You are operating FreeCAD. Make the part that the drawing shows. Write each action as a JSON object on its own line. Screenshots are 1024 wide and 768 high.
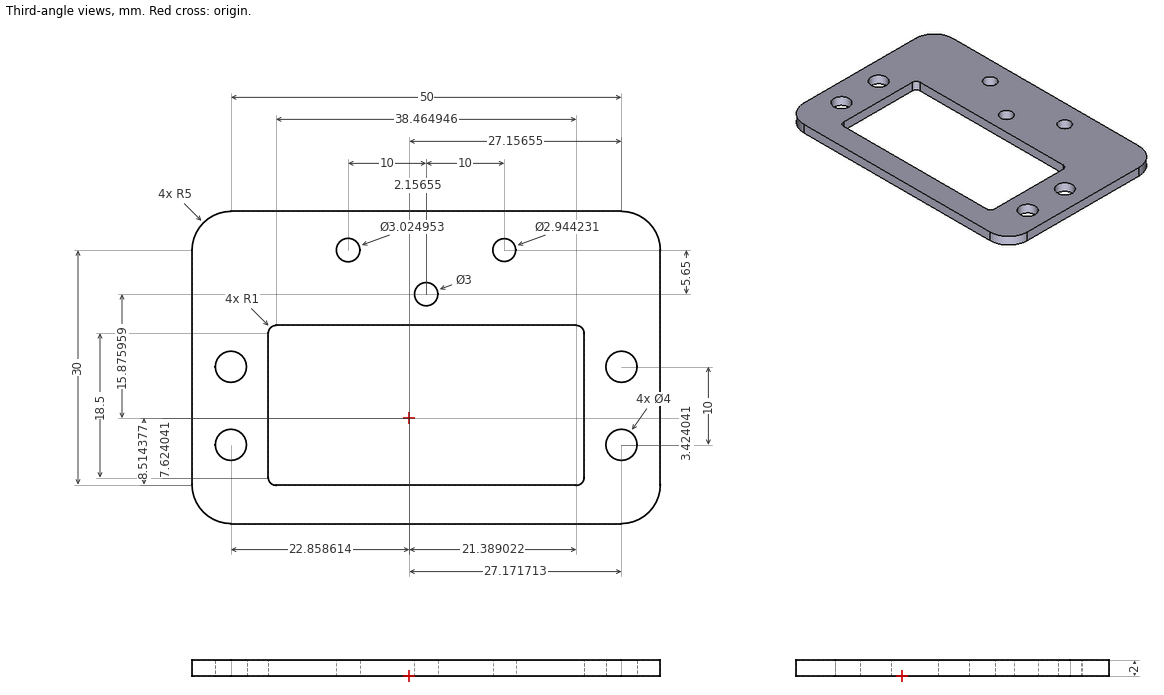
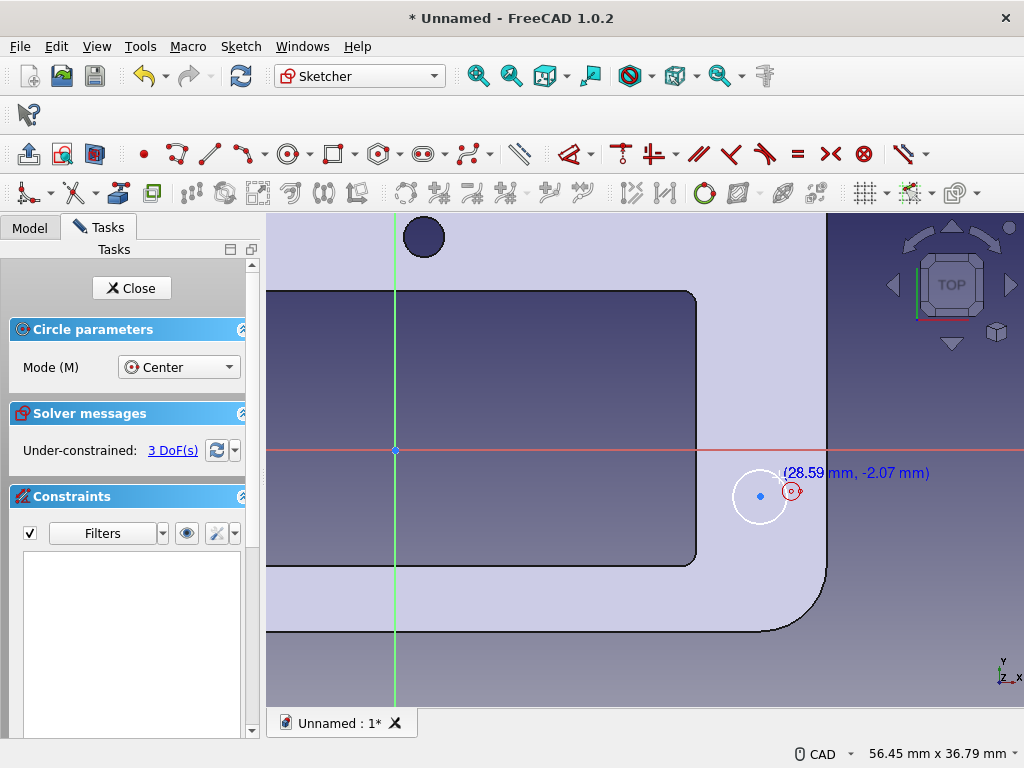
{"action": "left_click", "coordinate": [760, 362]}
{"action": "left_click", "coordinate": [779, 343]}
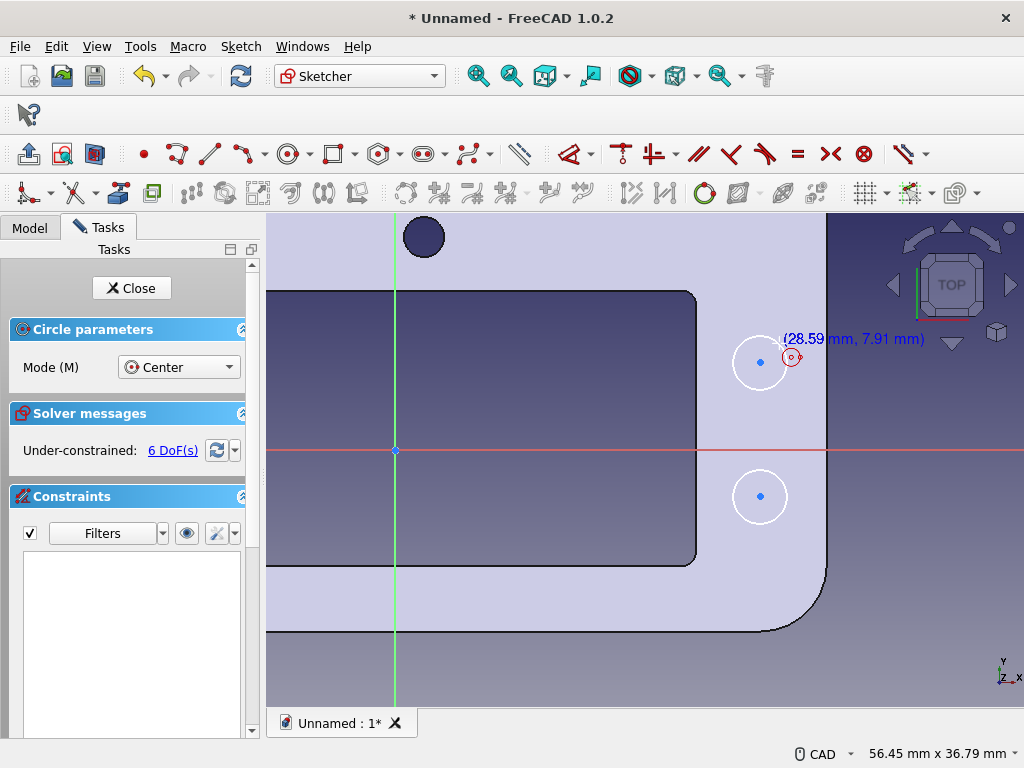
{"action": "scroll", "coordinate": [762, 498], "scroll_direction": "down", "scroll_amount": 3}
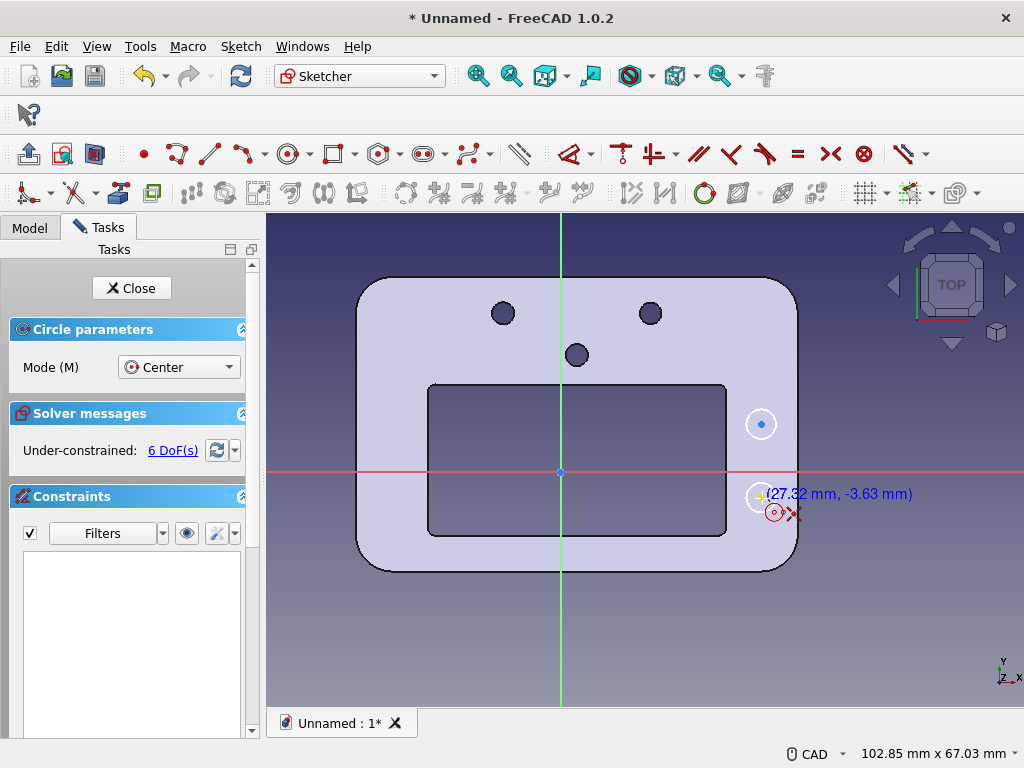
{"action": "scroll", "coordinate": [392, 497], "scroll_direction": "up", "scroll_amount": 3}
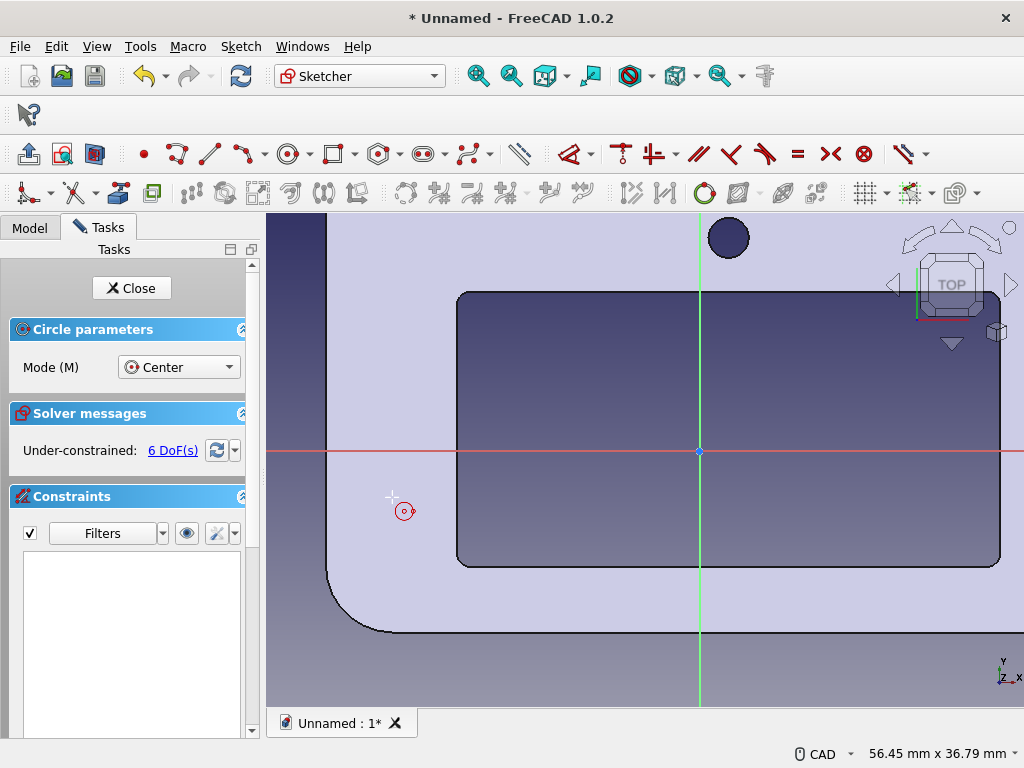
{"action": "left_click", "coordinate": [393, 497]}
{"action": "left_click", "coordinate": [412, 478]}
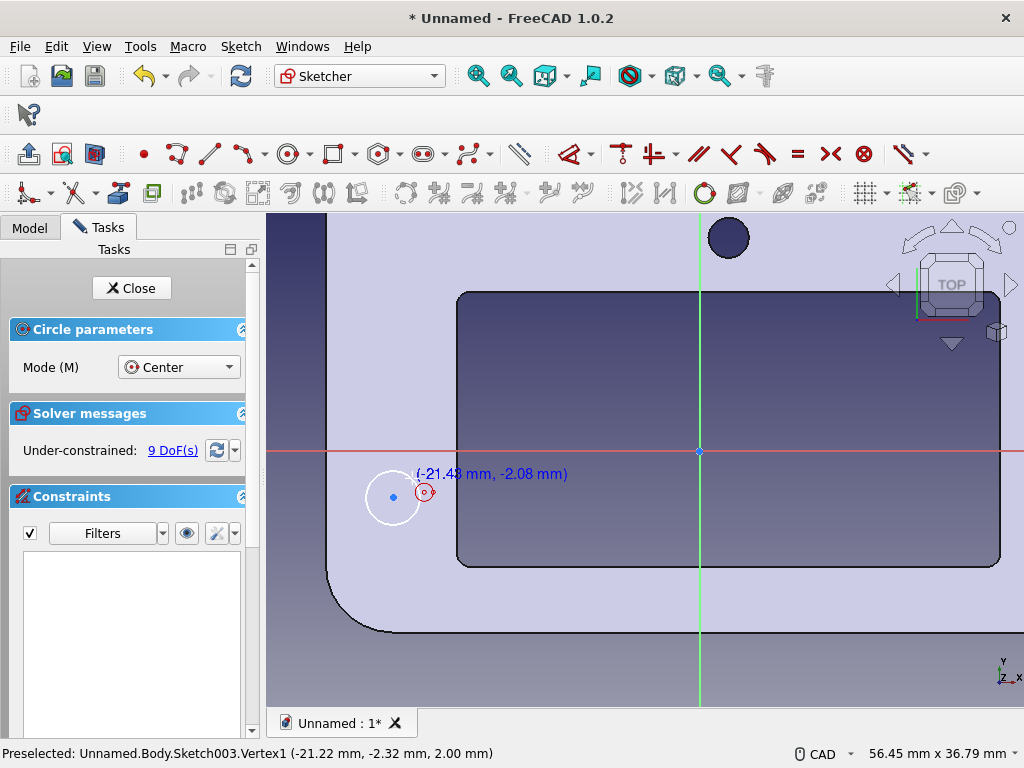
{"action": "left_click", "coordinate": [393, 363]}
{"action": "left_click", "coordinate": [412, 344]}
{"action": "key", "text": "Escape"}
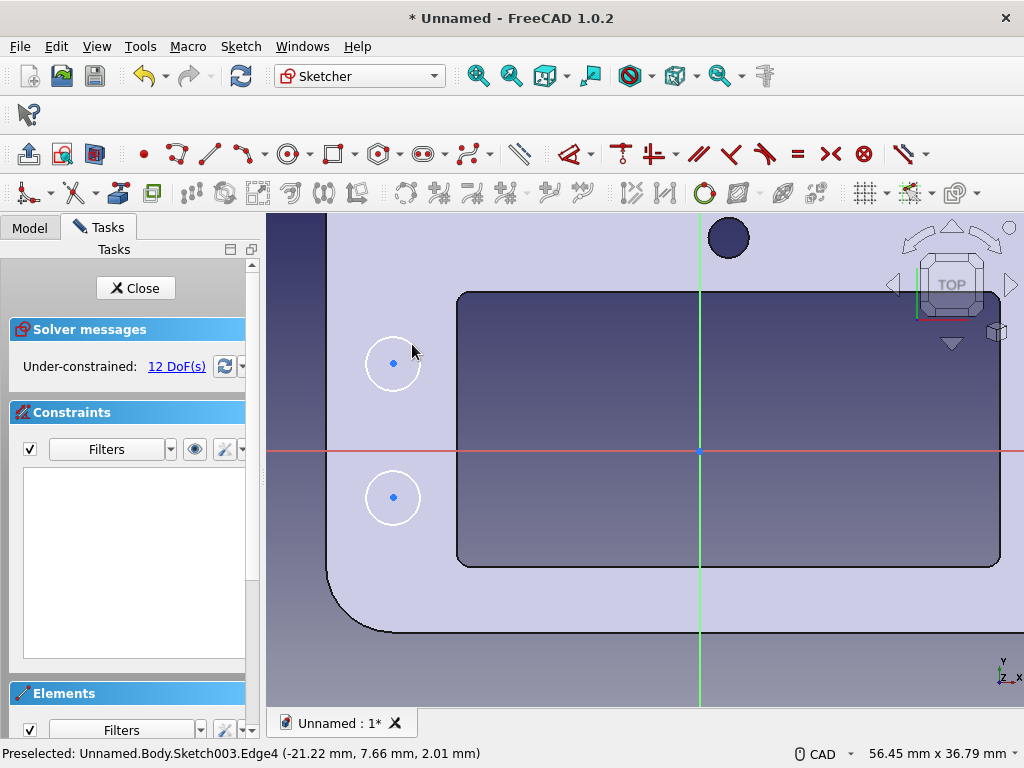
{"action": "scroll", "coordinate": [391, 497], "scroll_direction": "down", "scroll_amount": 3}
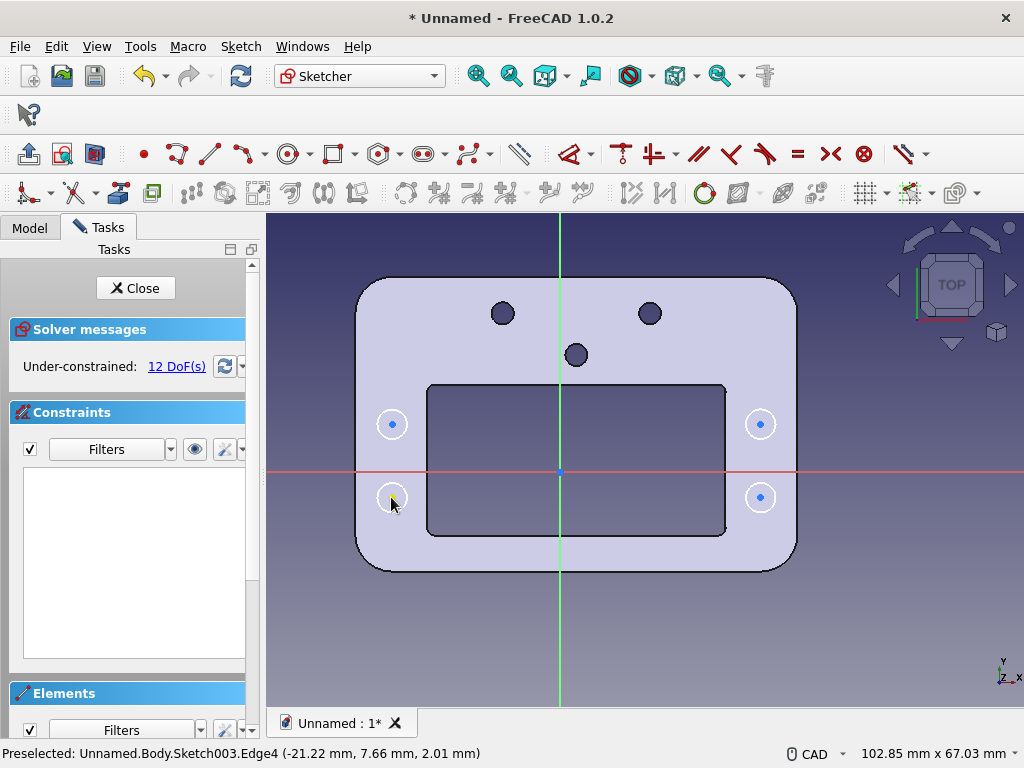
{"action": "left_click", "coordinate": [771, 487]}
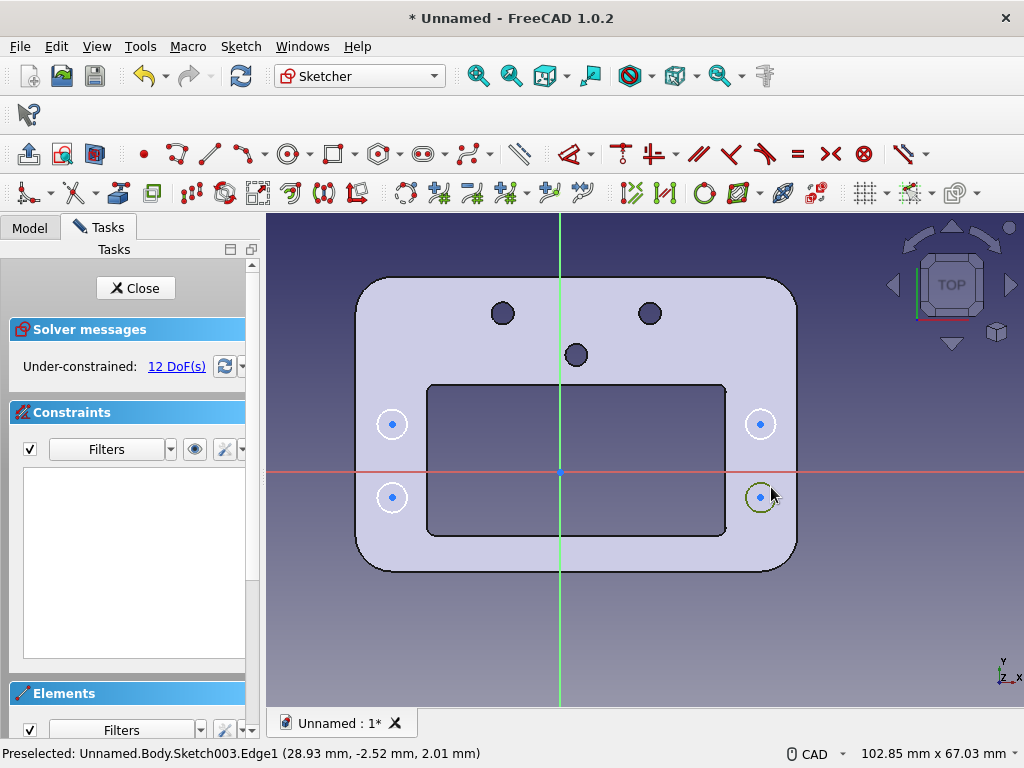
{"action": "left_click", "coordinate": [771, 414]}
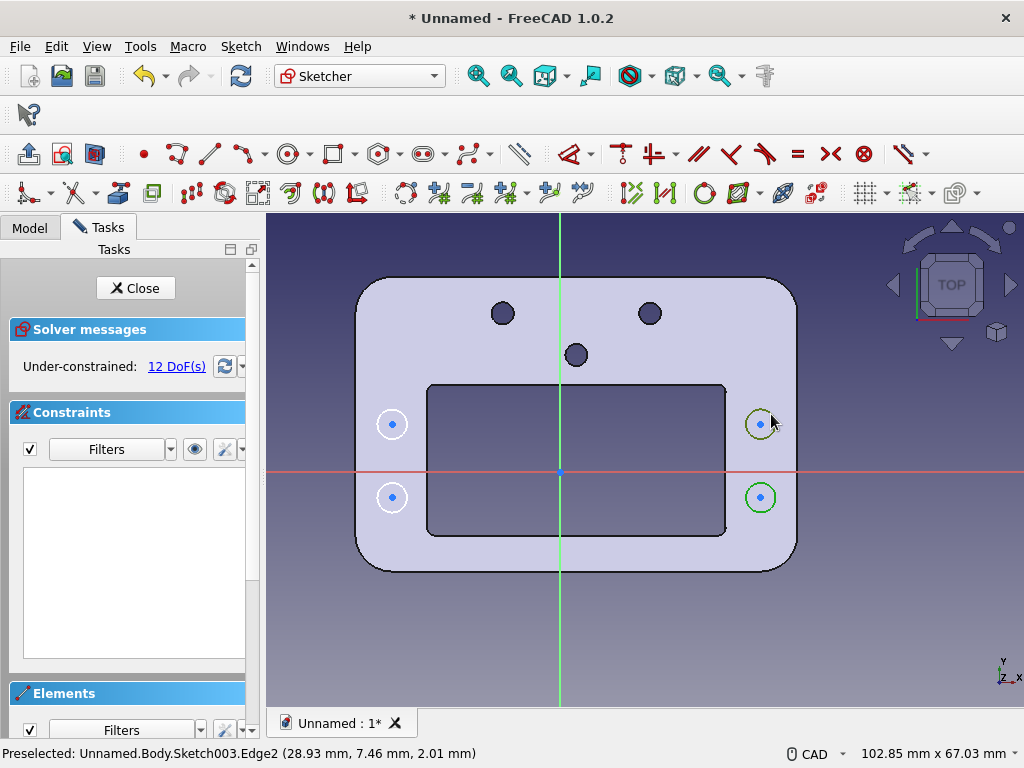
{"action": "left_click", "coordinate": [403, 487]}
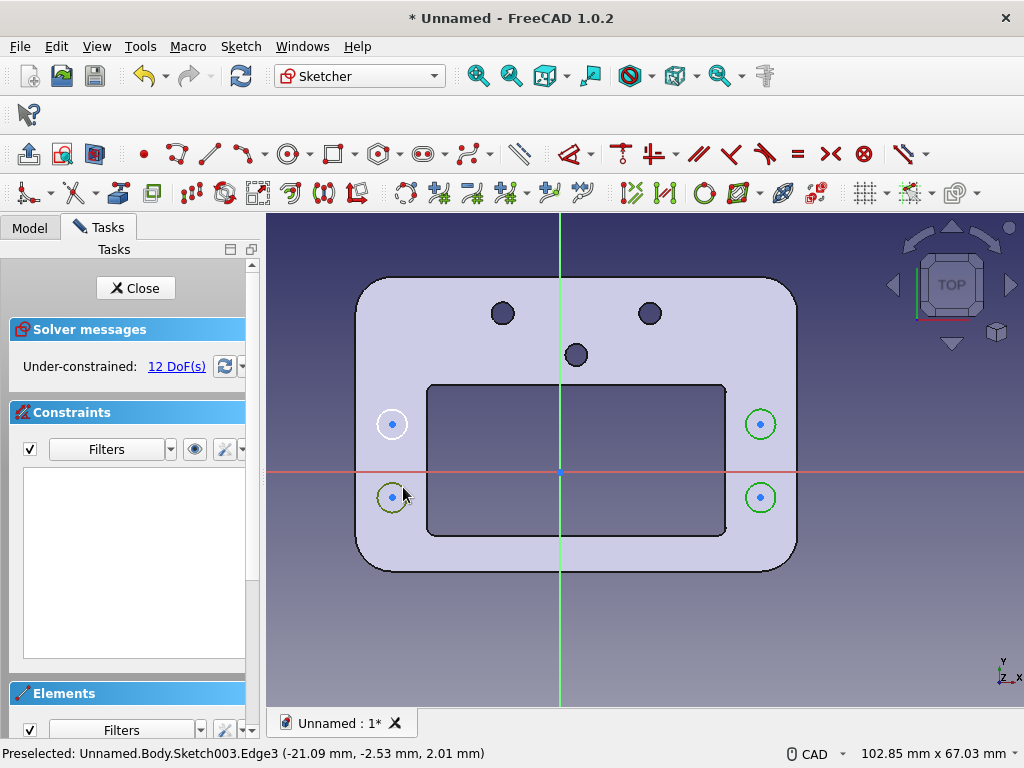
{"action": "left_click", "coordinate": [403, 414]}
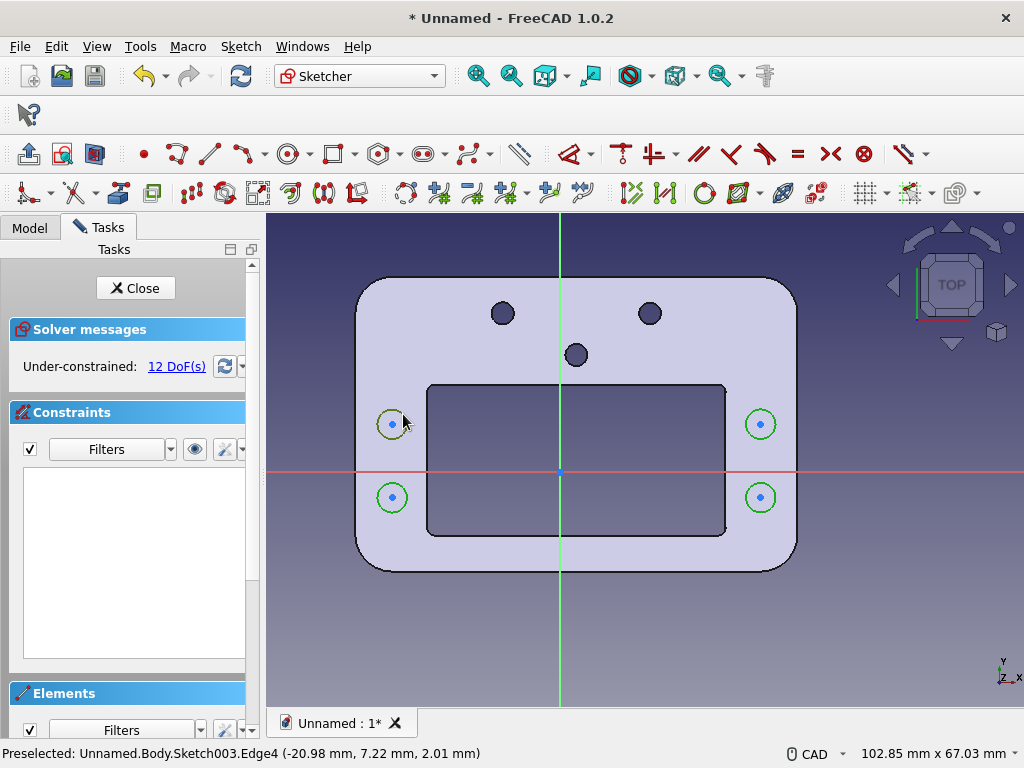
{"action": "left_click", "coordinate": [798, 154]}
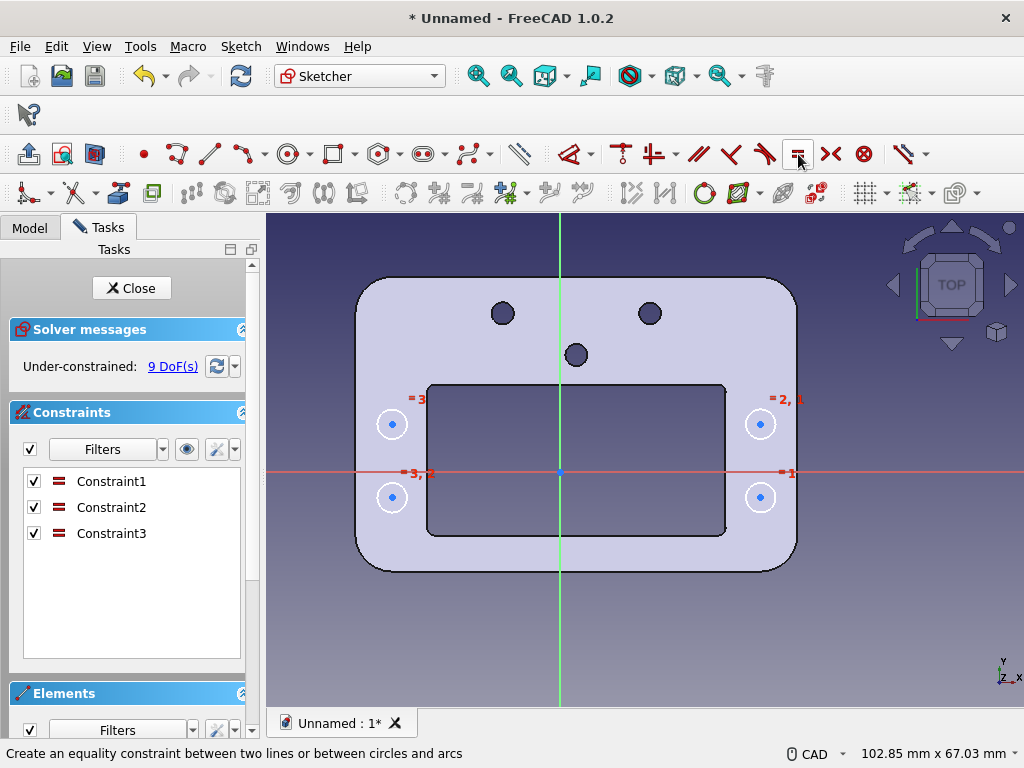
{"action": "left_click", "coordinate": [568, 154]}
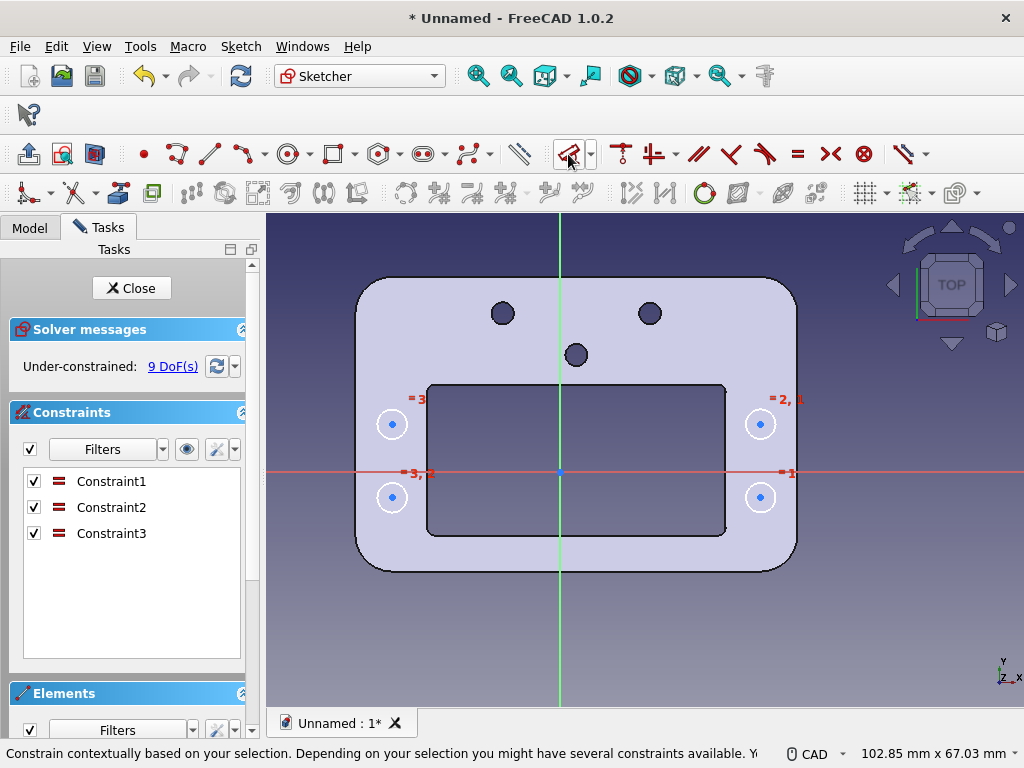
{"action": "scroll", "coordinate": [771, 487], "scroll_direction": "up", "scroll_amount": 2}